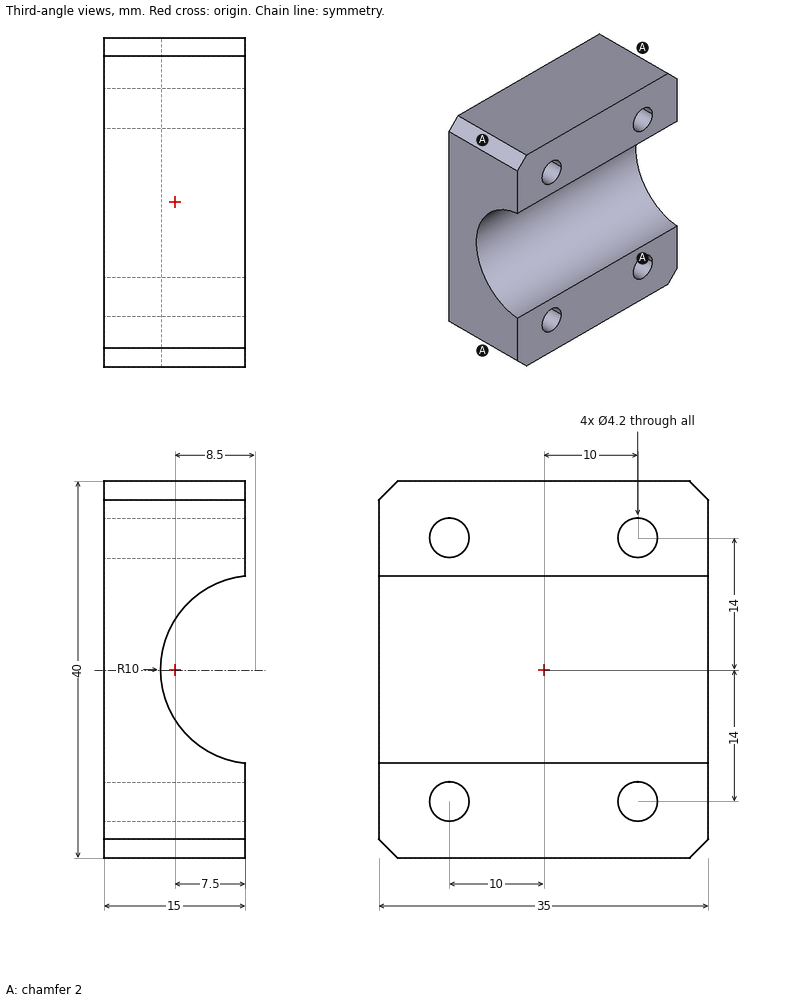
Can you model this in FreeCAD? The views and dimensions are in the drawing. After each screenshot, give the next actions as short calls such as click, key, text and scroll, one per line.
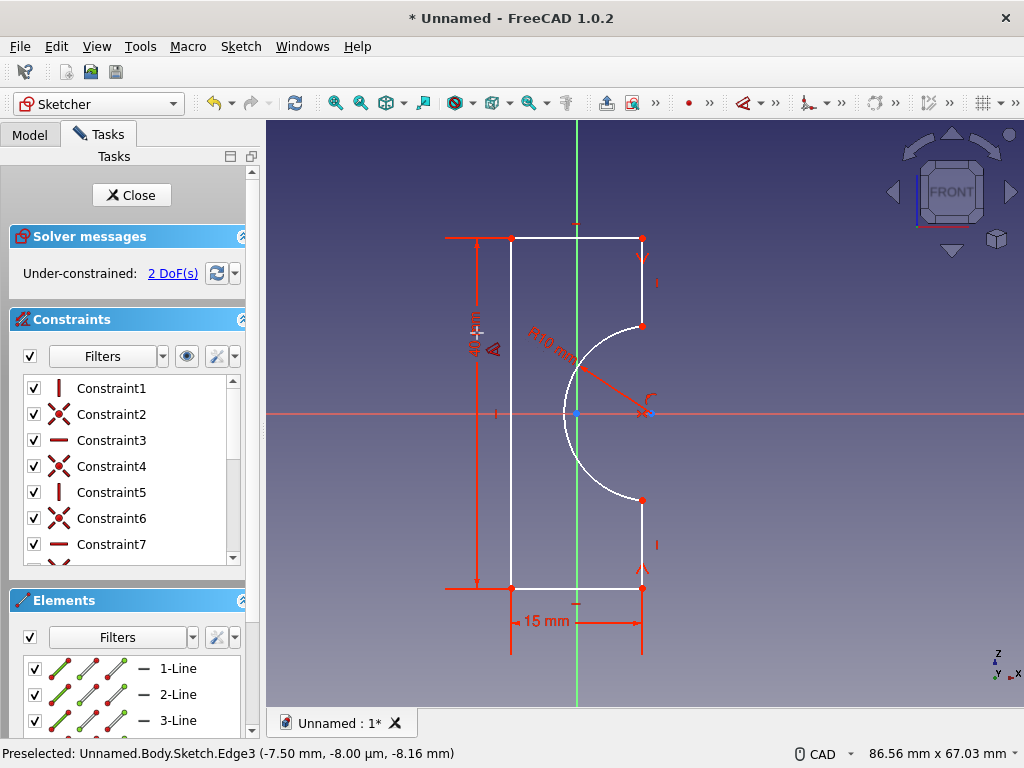
click(642, 501)
click(610, 535)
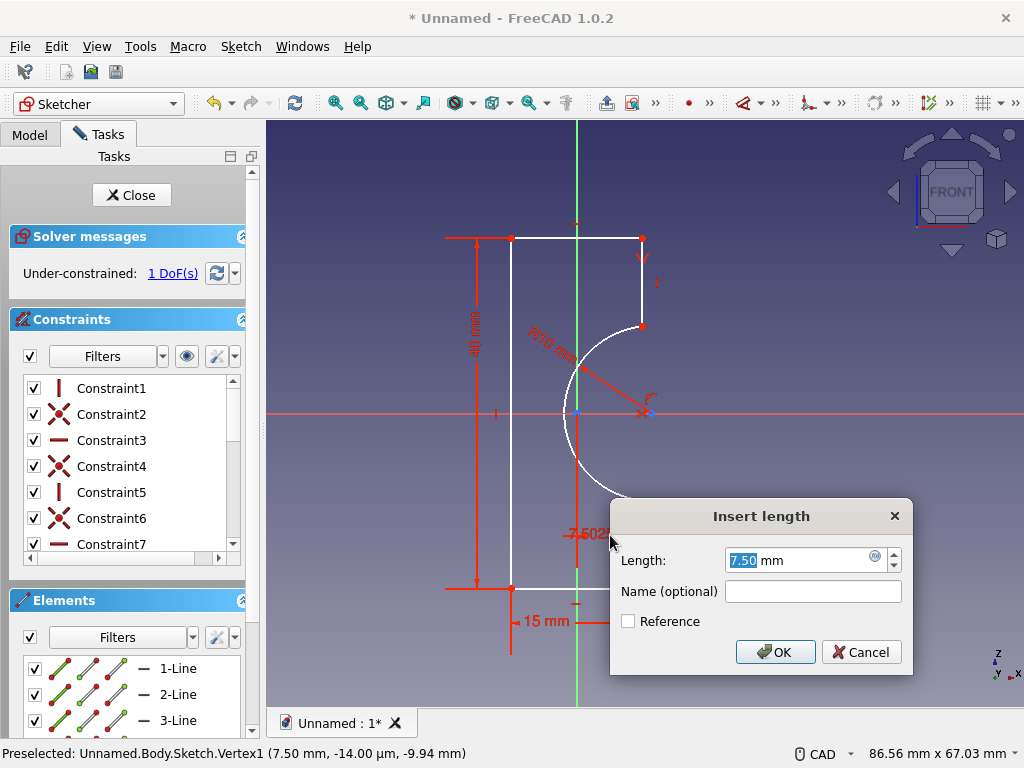
text(7.5)
key(Return)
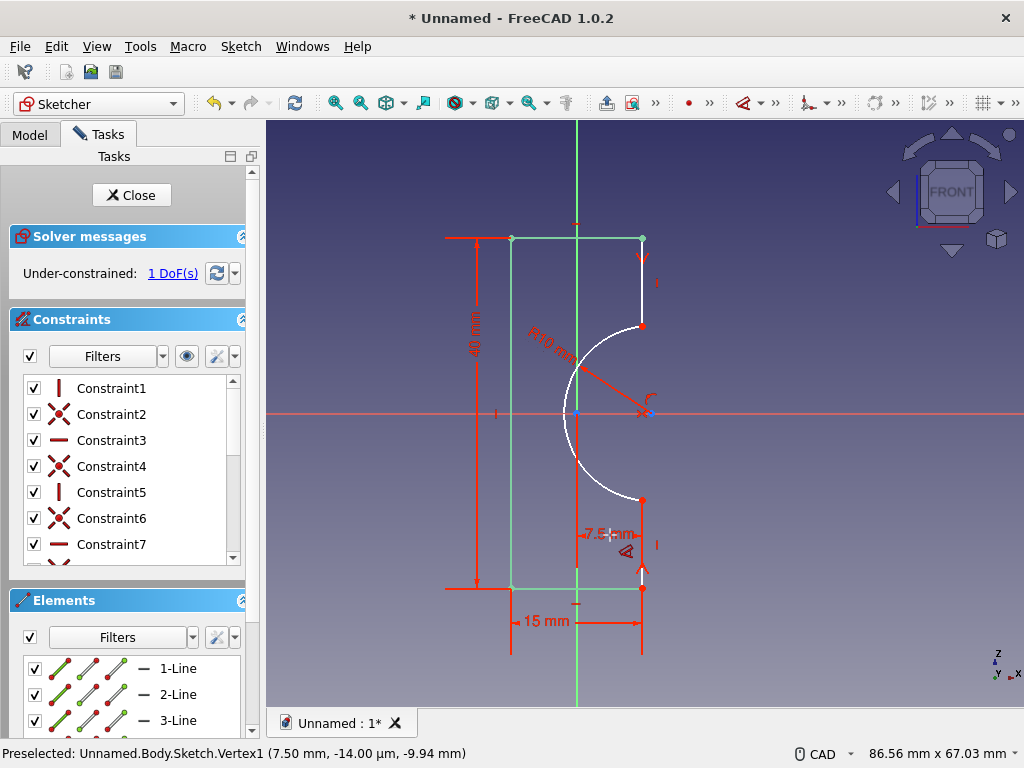
click(652, 413)
click(614, 447)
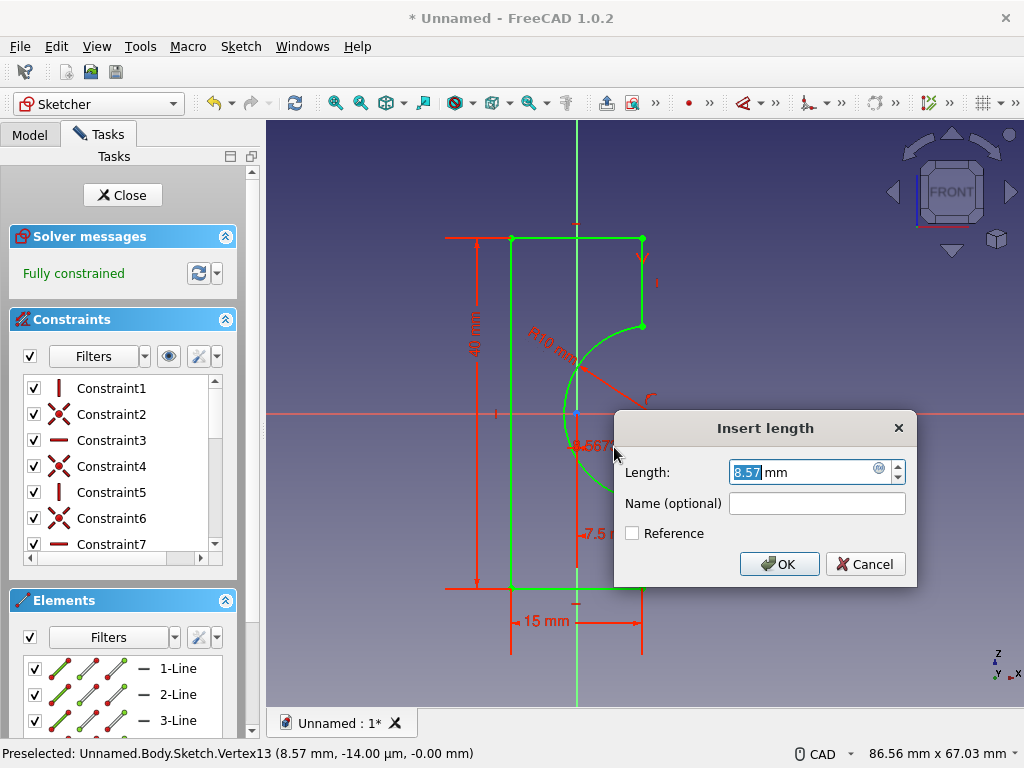
text(8.5)
key(Return)
key(Escape)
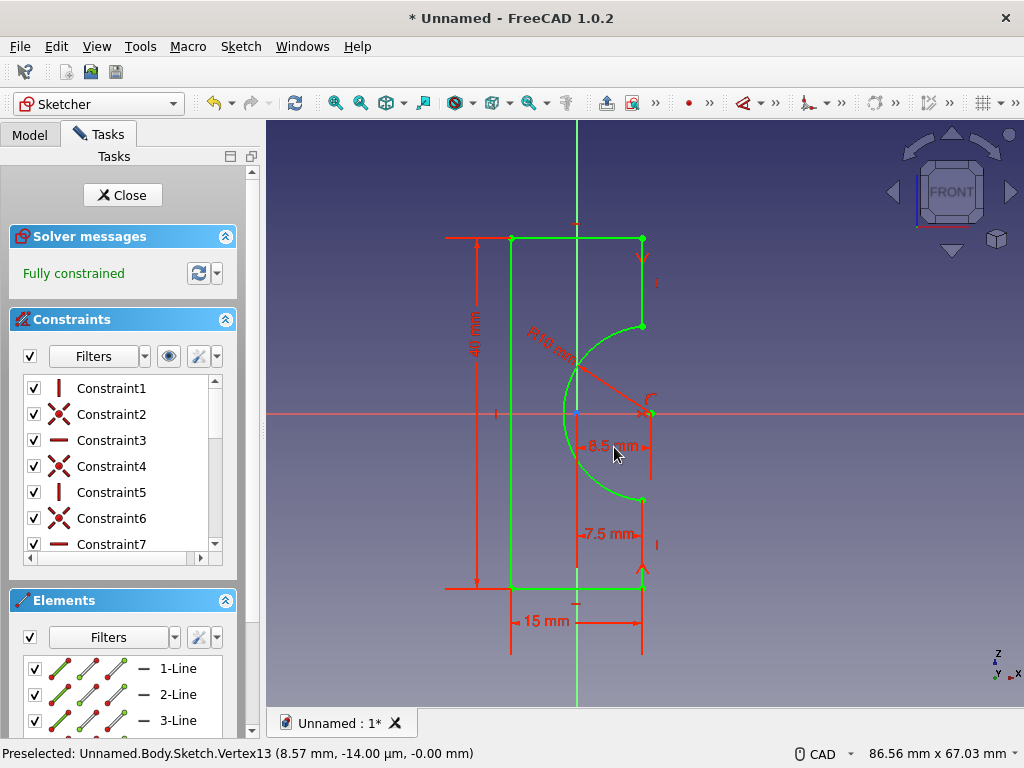
click(123, 195)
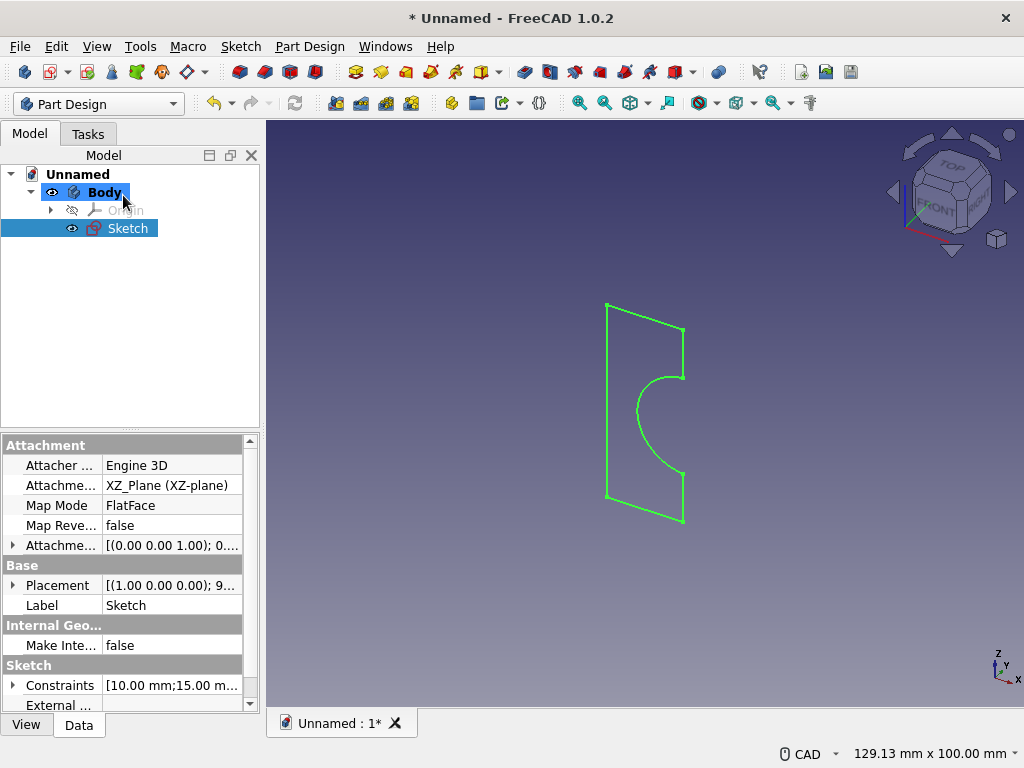
click(356, 72)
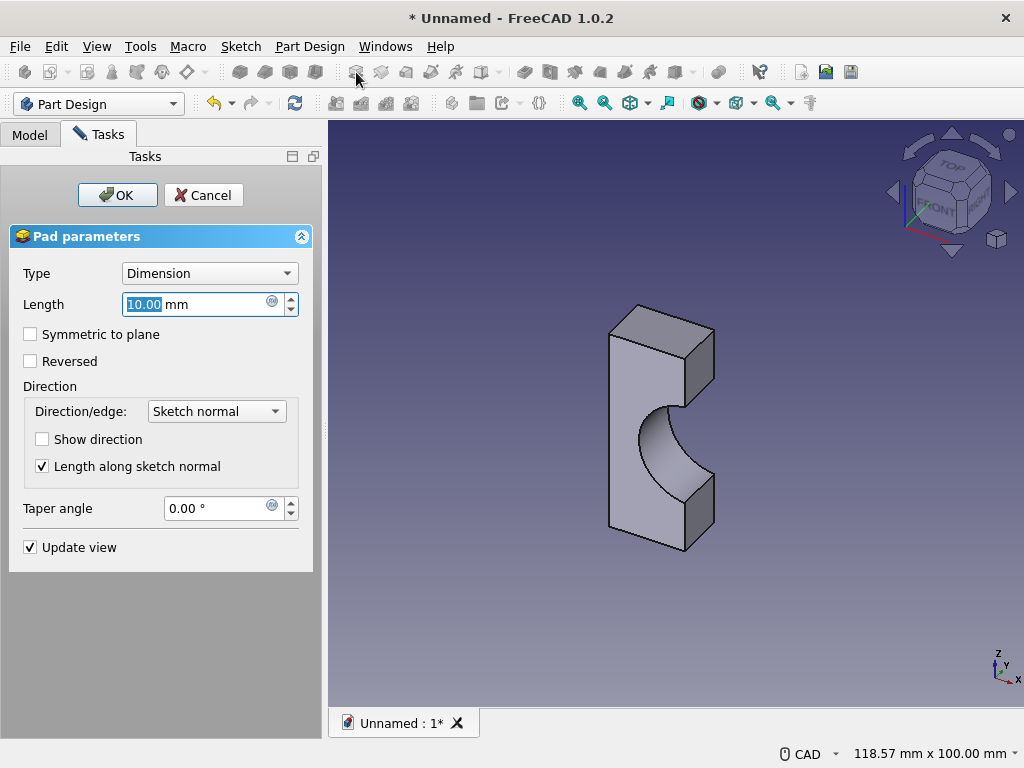
text(35)
key(Tab)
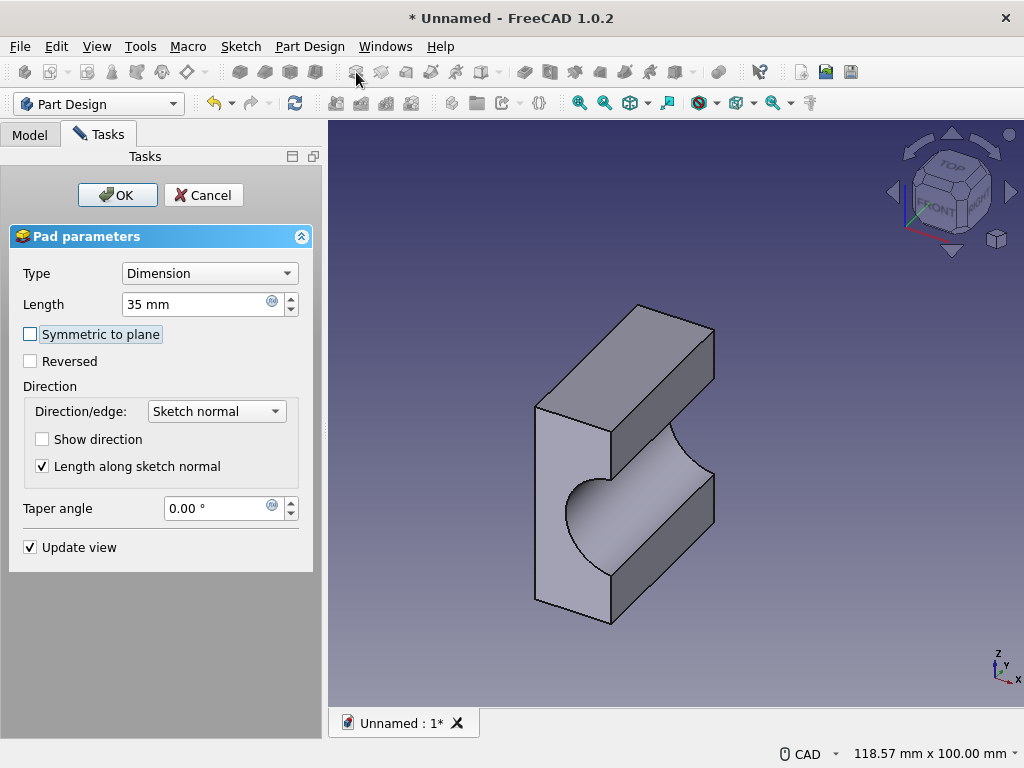
click(31, 334)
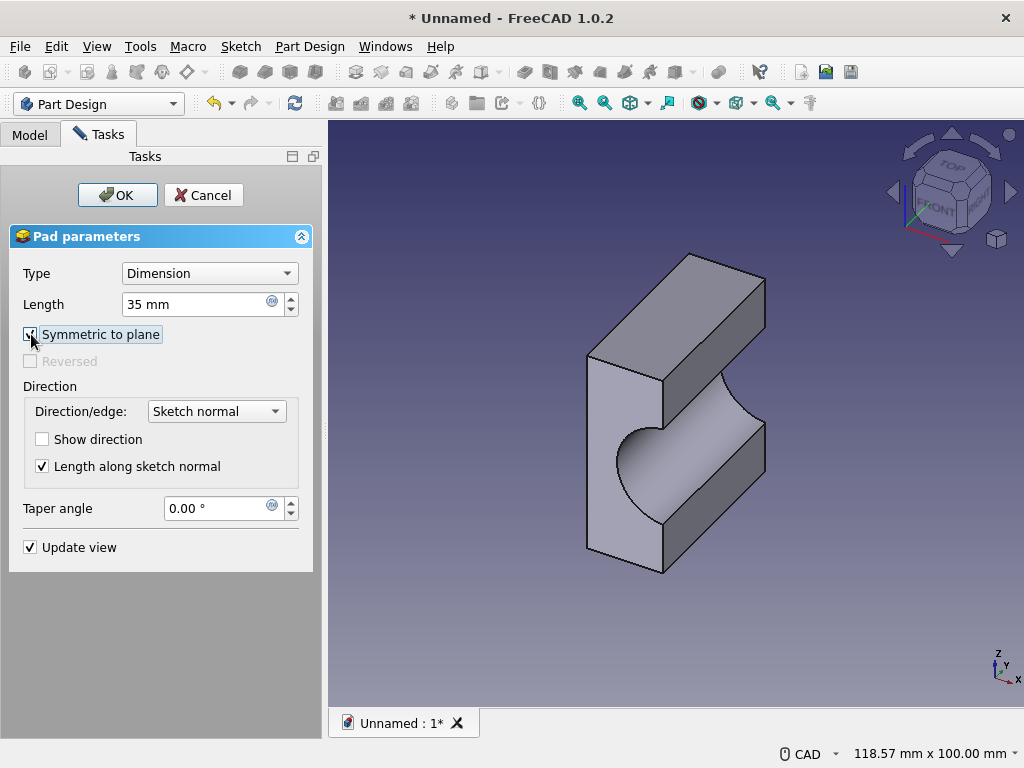
click(118, 195)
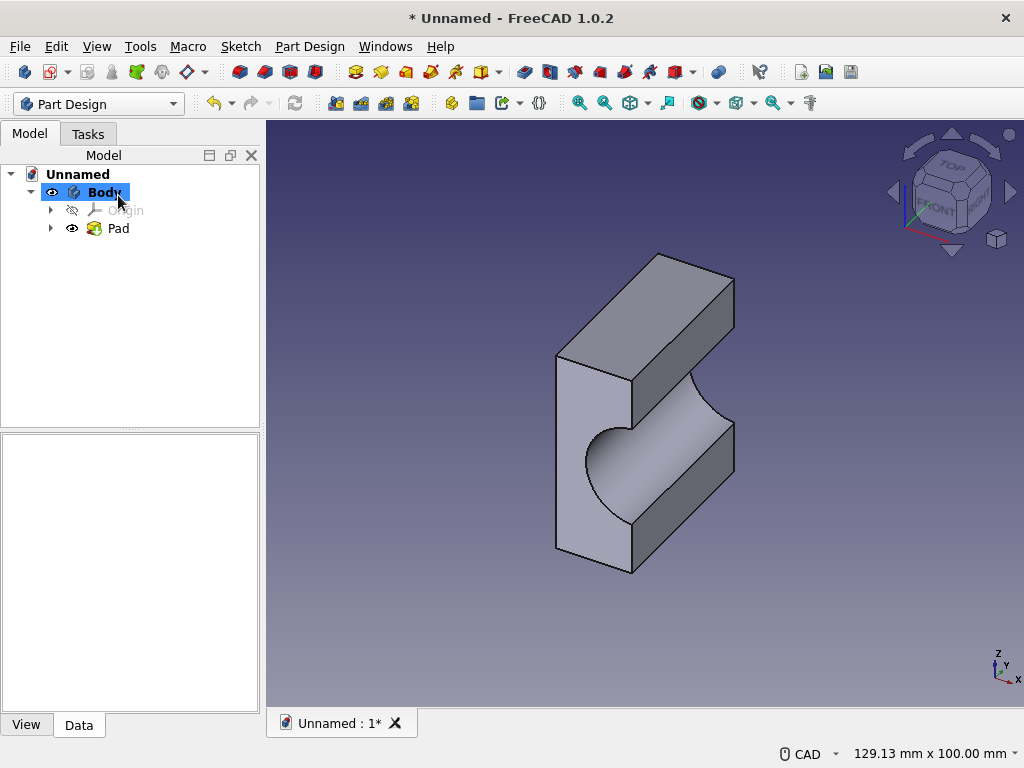
click(594, 367)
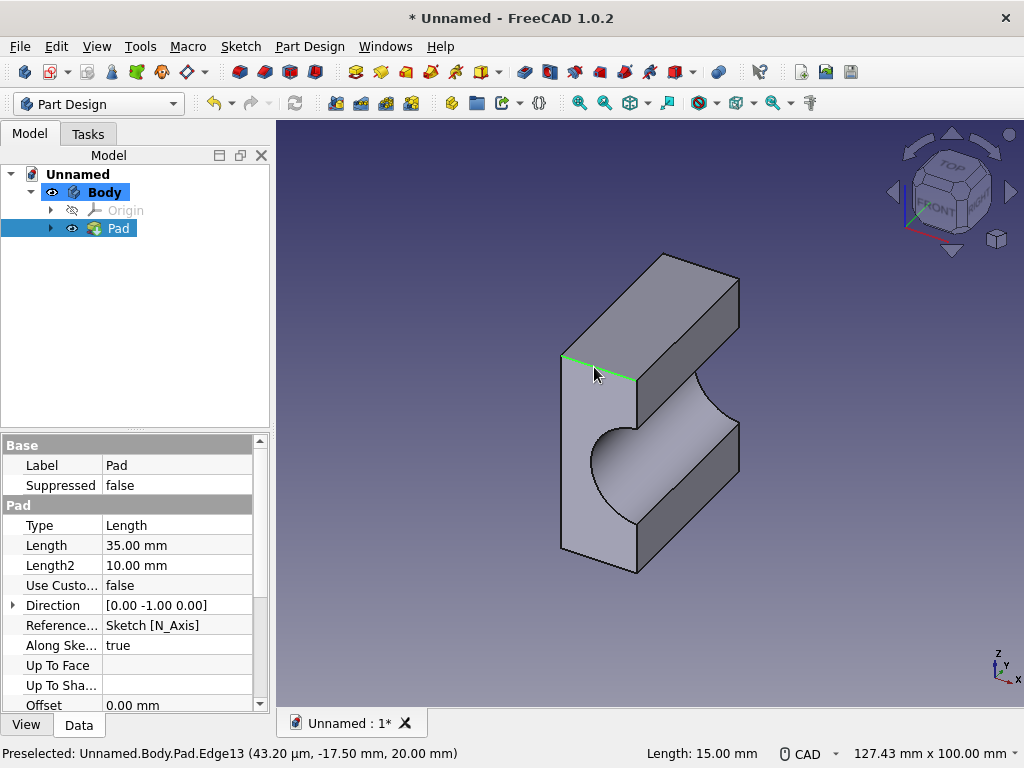
key(0)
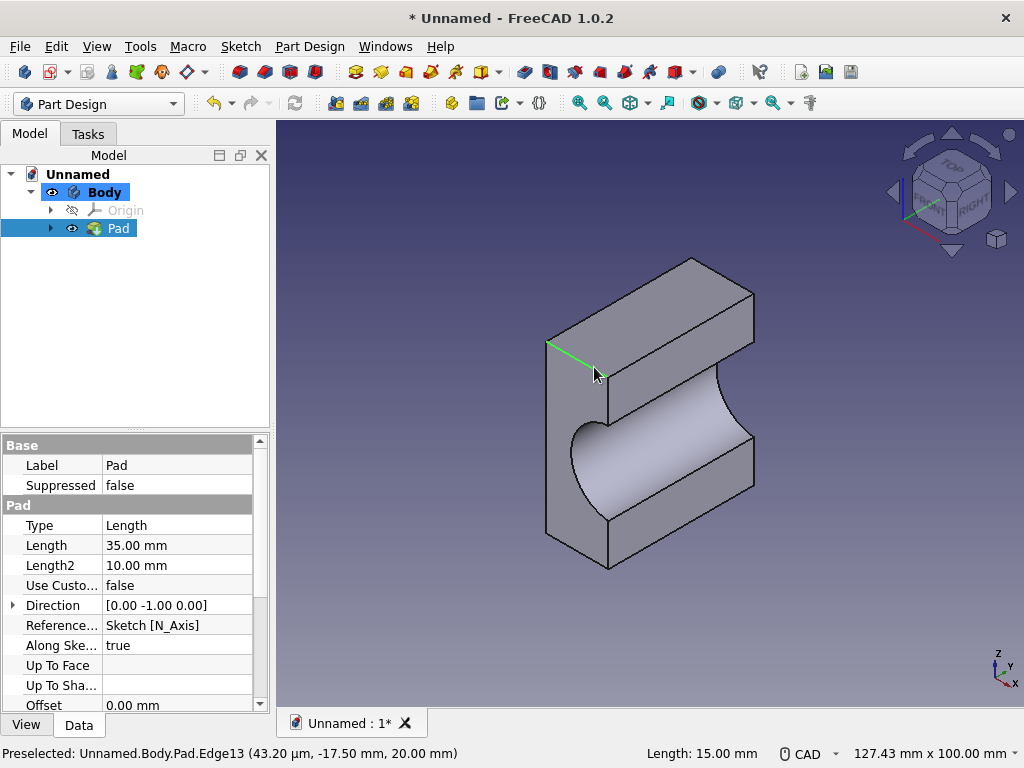
key(2)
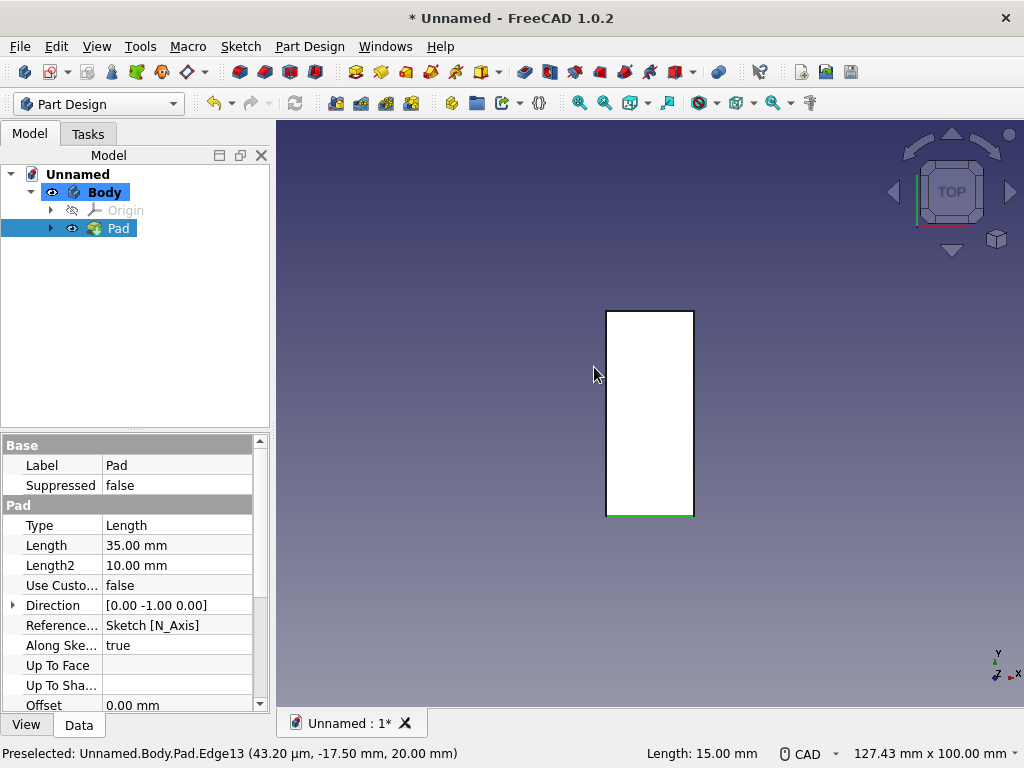
click(580, 104)